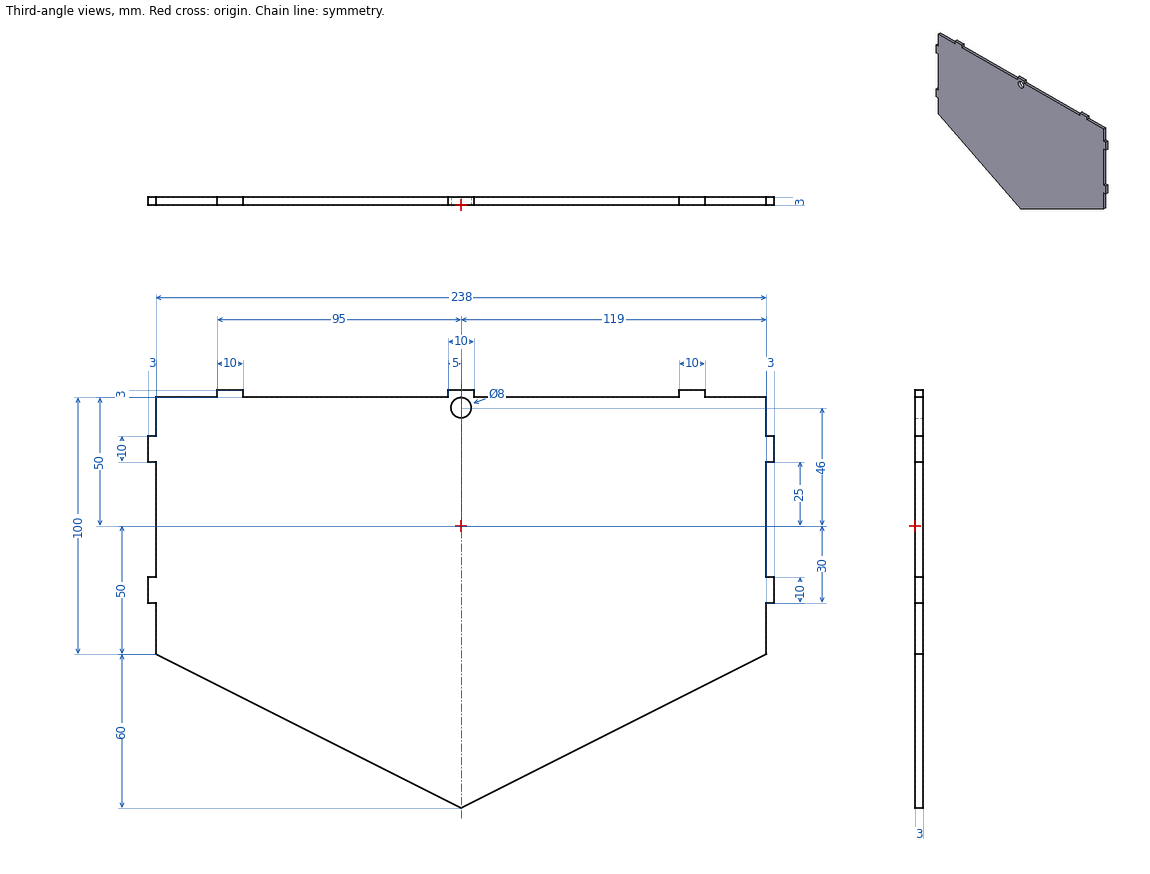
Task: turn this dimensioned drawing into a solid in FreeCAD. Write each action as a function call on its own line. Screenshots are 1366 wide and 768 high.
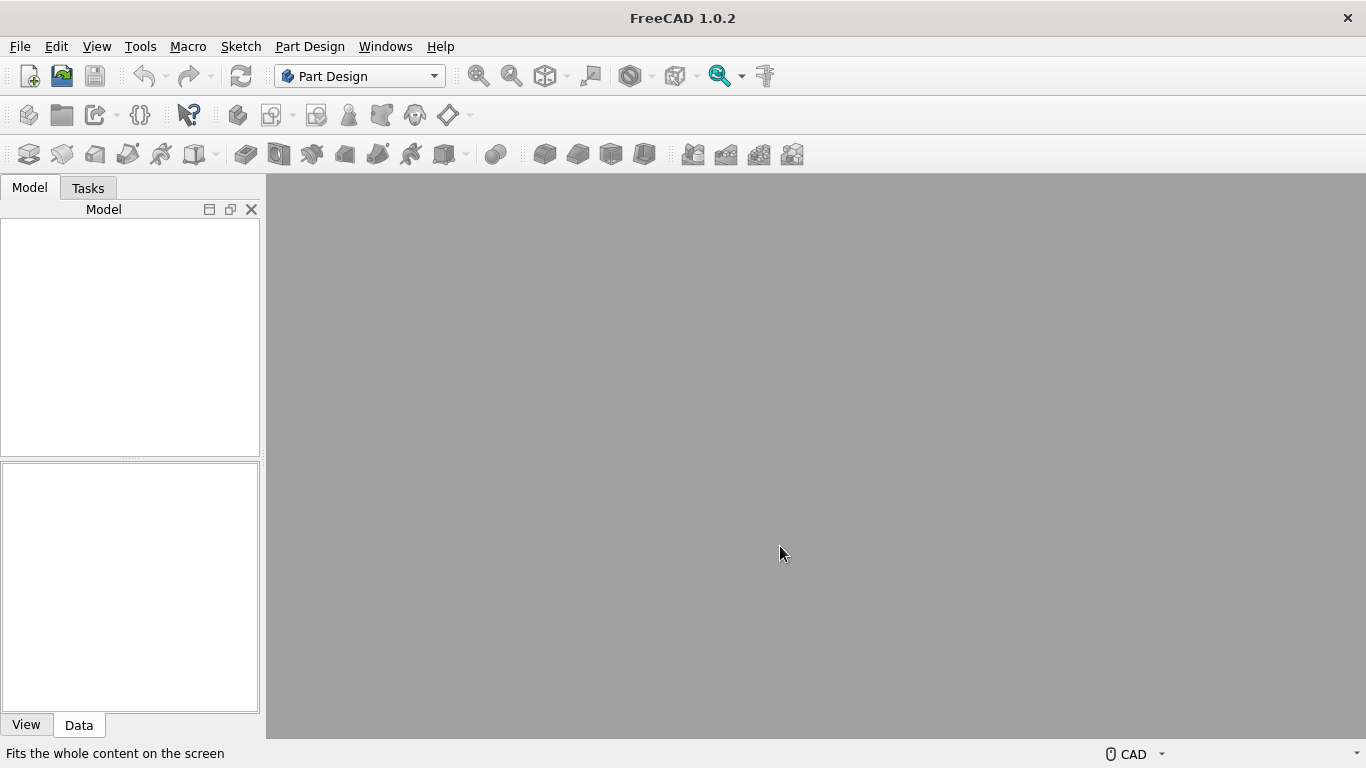
click(29, 76)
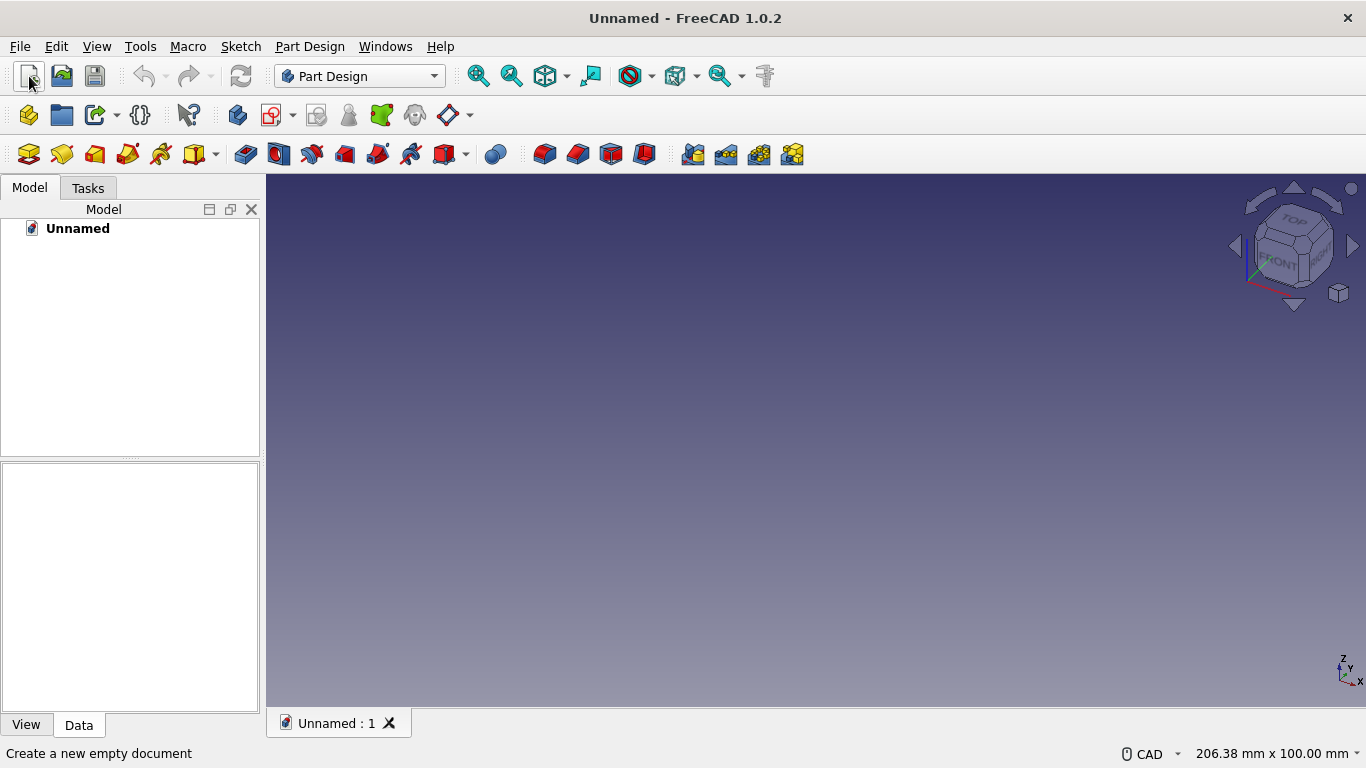
click(270, 116)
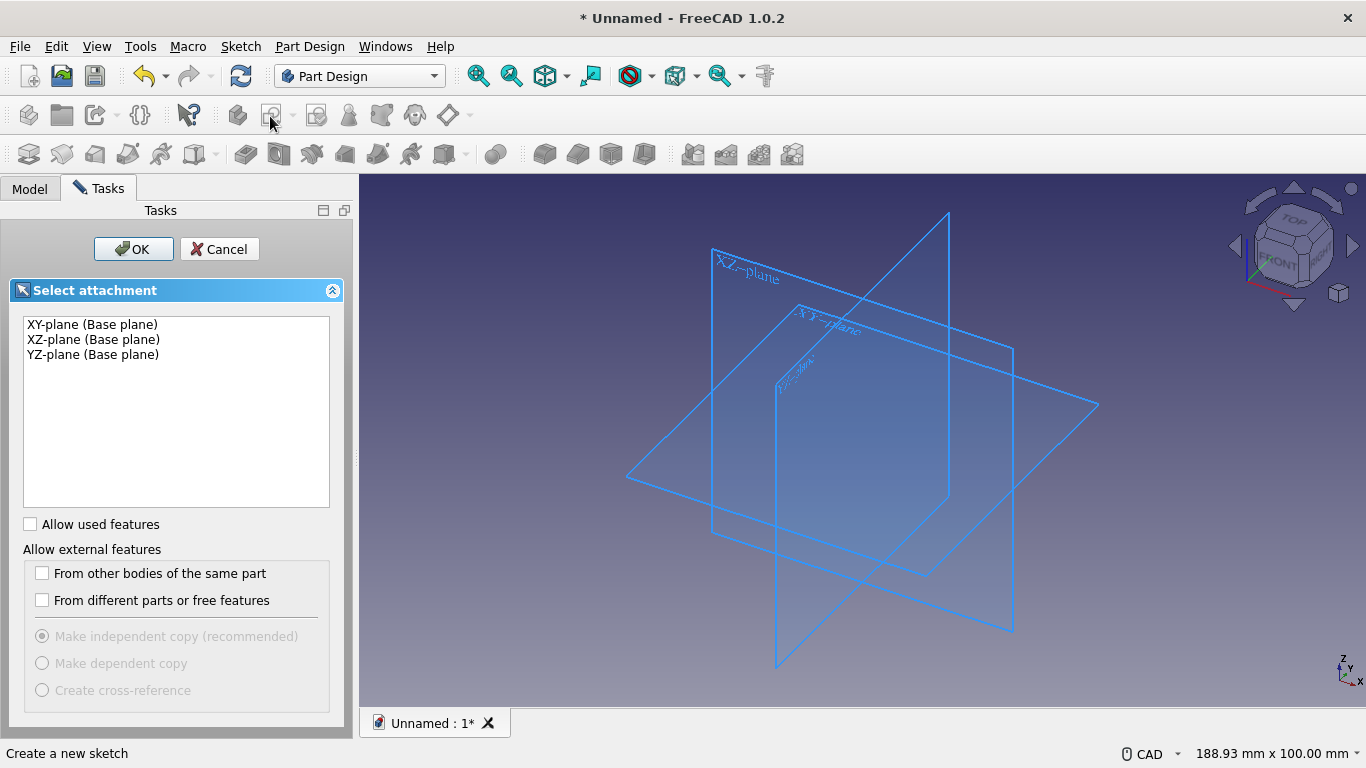
click(84, 340)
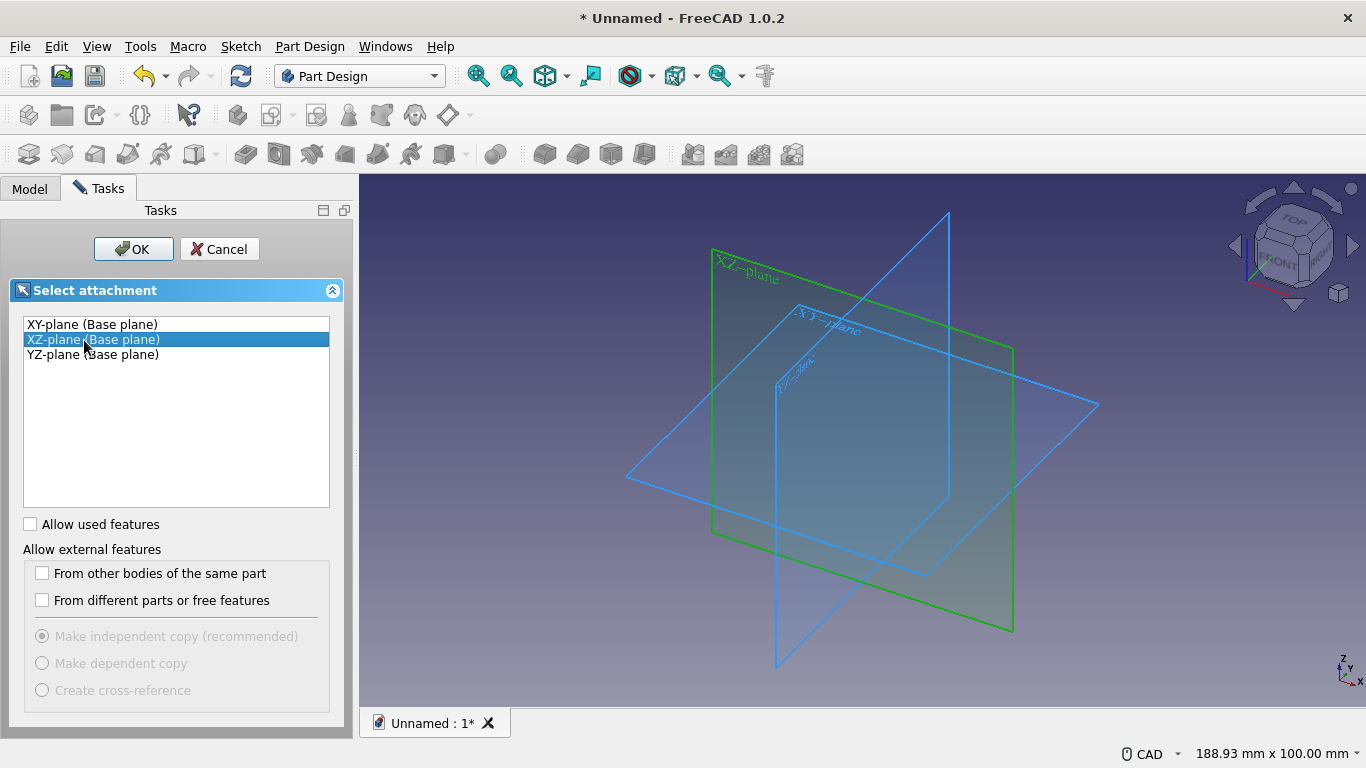
click(134, 249)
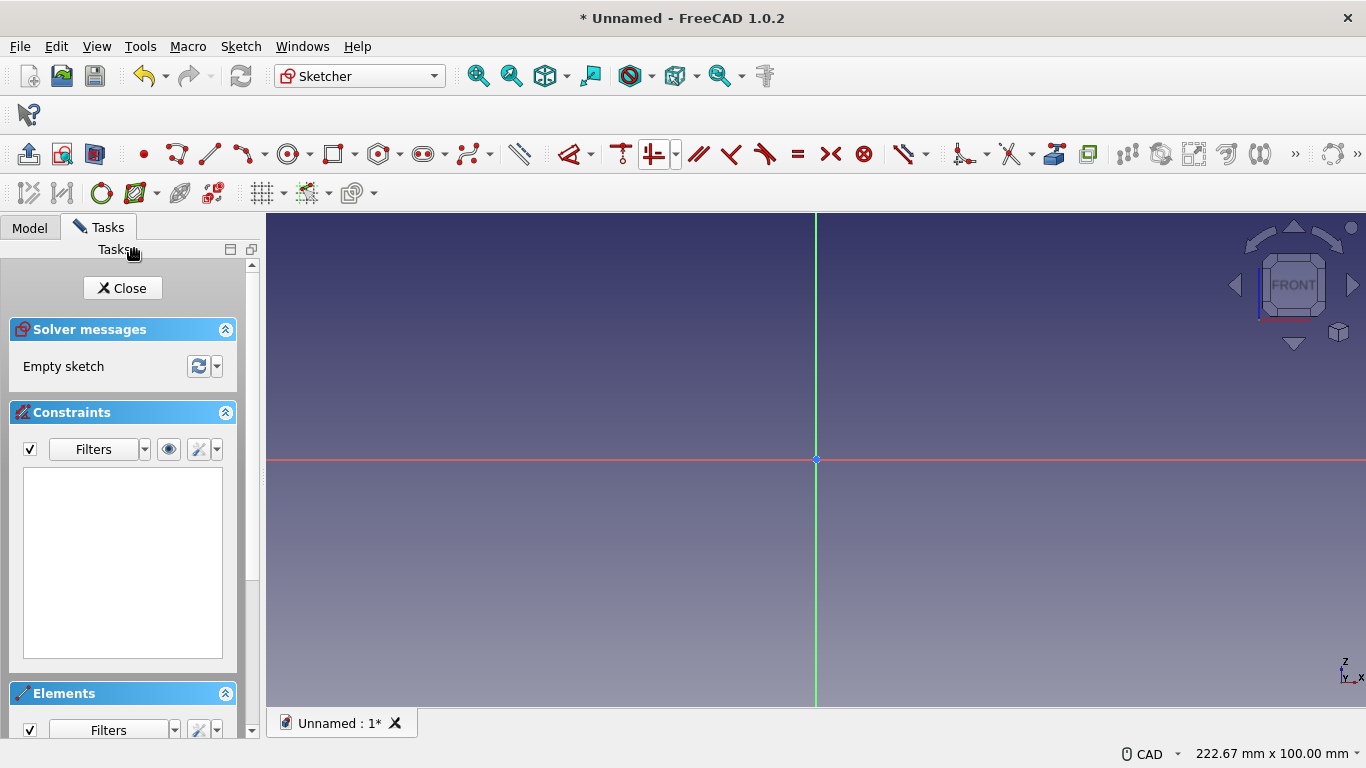
scroll(708, 374, down, 5)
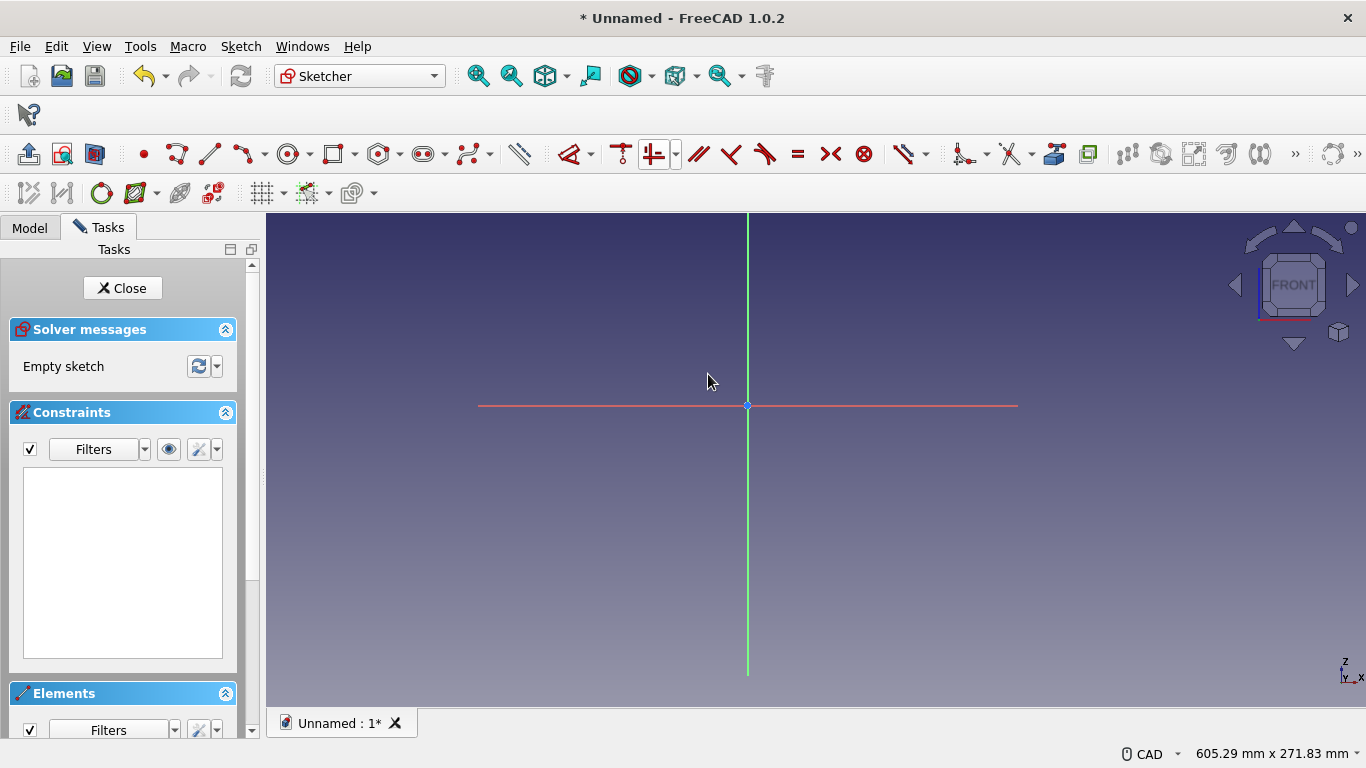
click(177, 154)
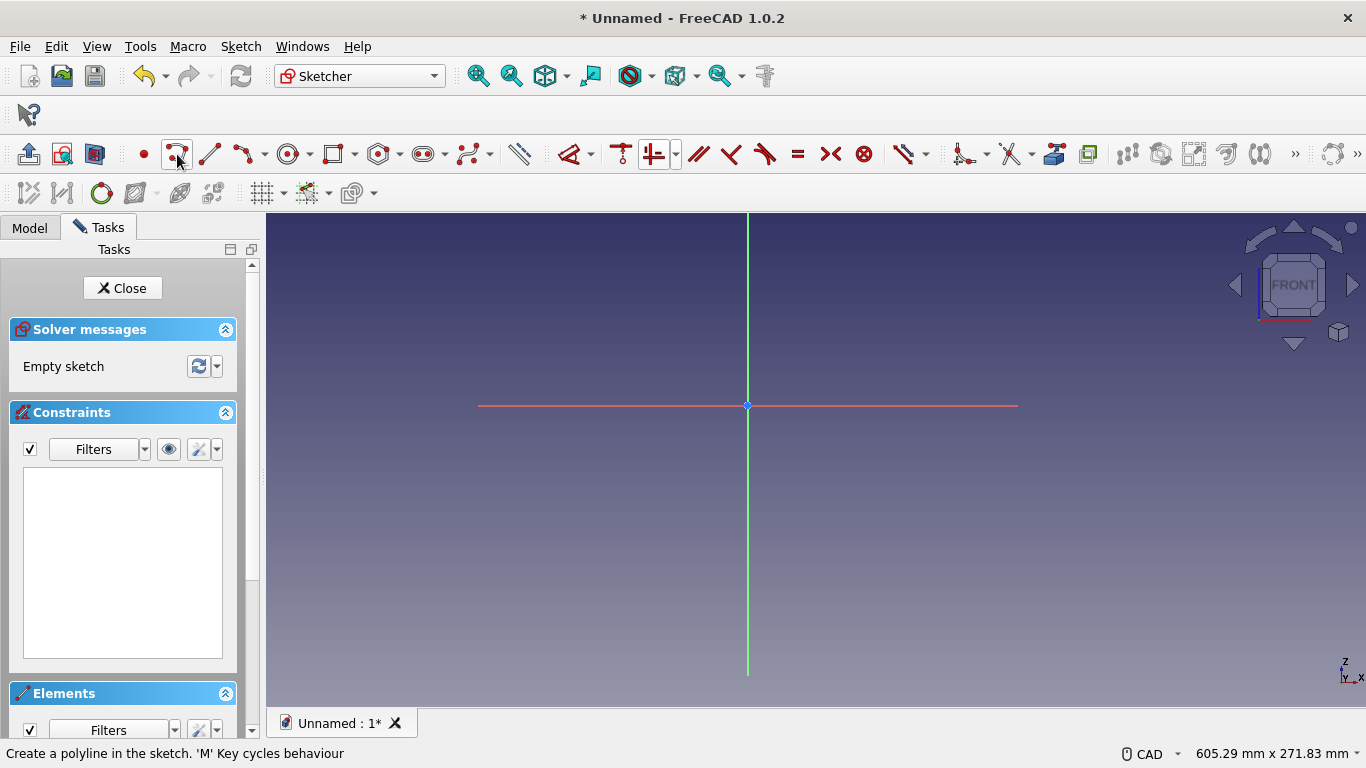
click(748, 606)
click(532, 497)
click(532, 315)
click(964, 315)
click(964, 497)
click(748, 607)
key(Escape)
key(Escape)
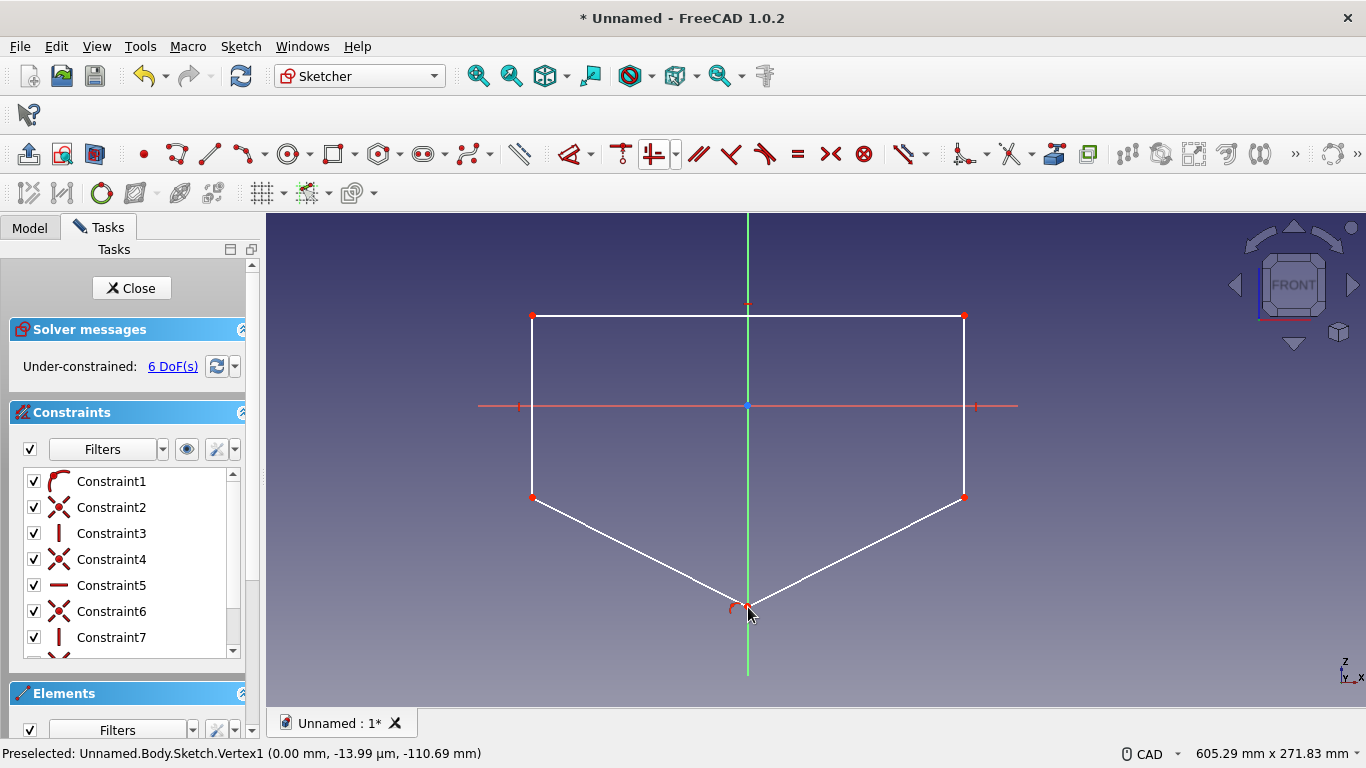
click(532, 498)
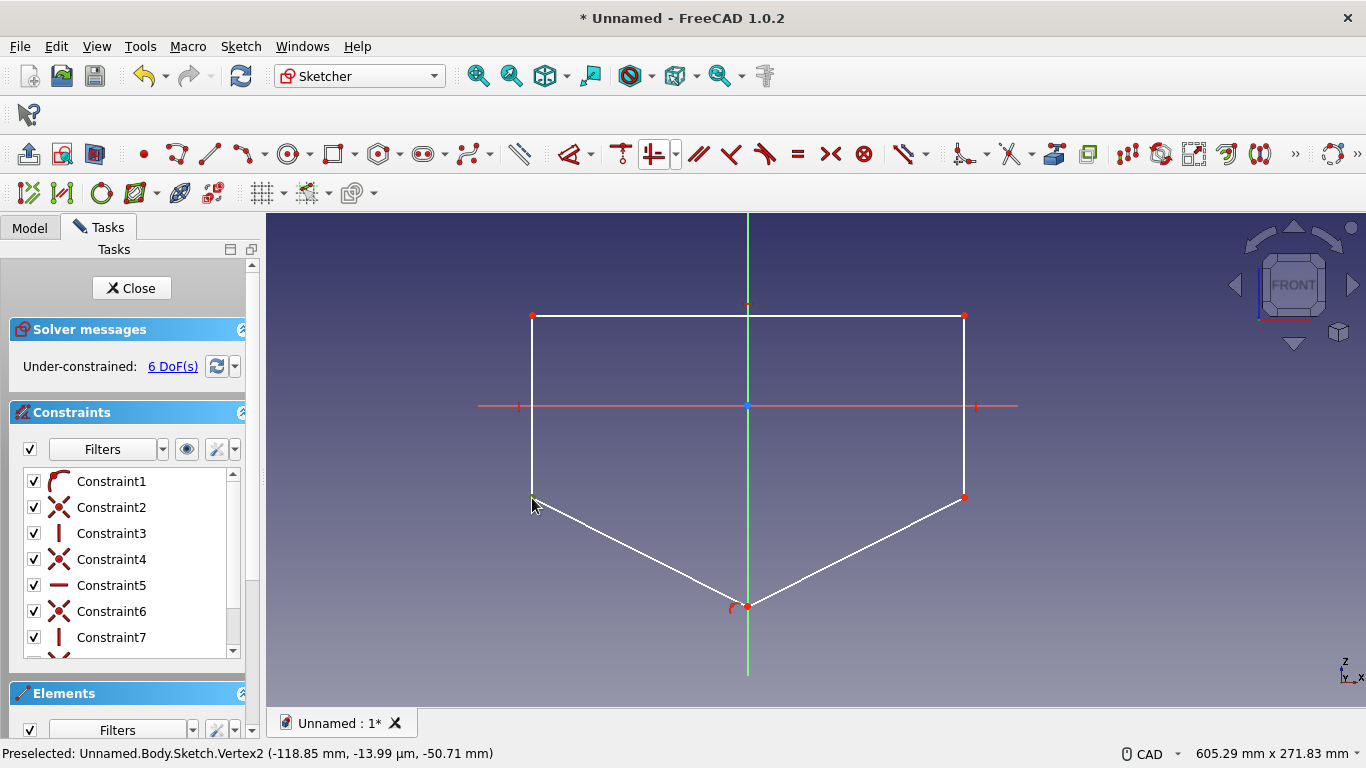
click(964, 498)